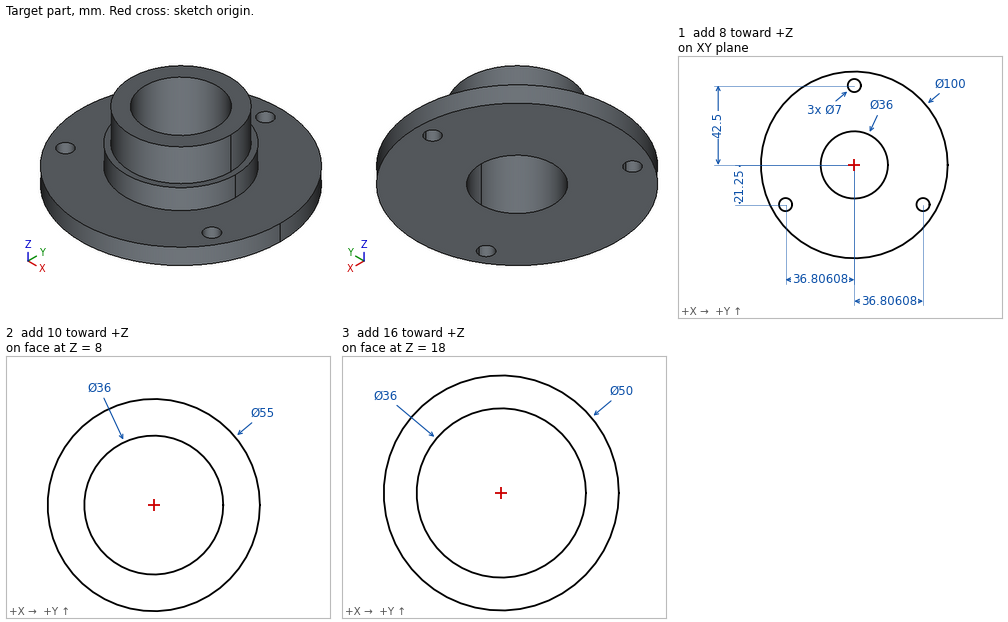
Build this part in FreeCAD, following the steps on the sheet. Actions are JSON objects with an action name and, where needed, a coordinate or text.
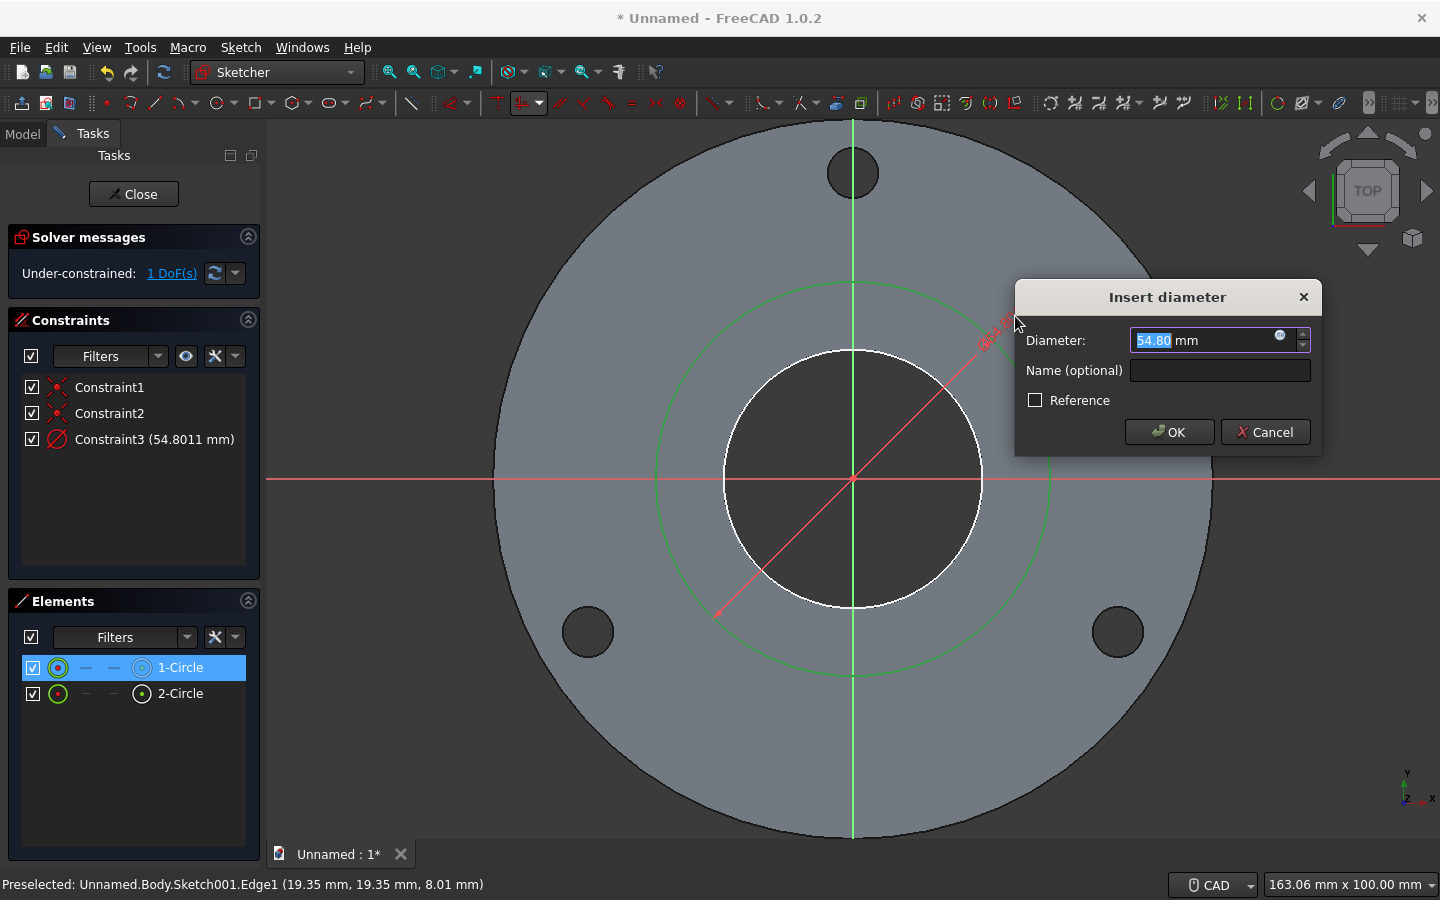
{"action": "type", "text": "55"}
{"action": "key", "text": "Return"}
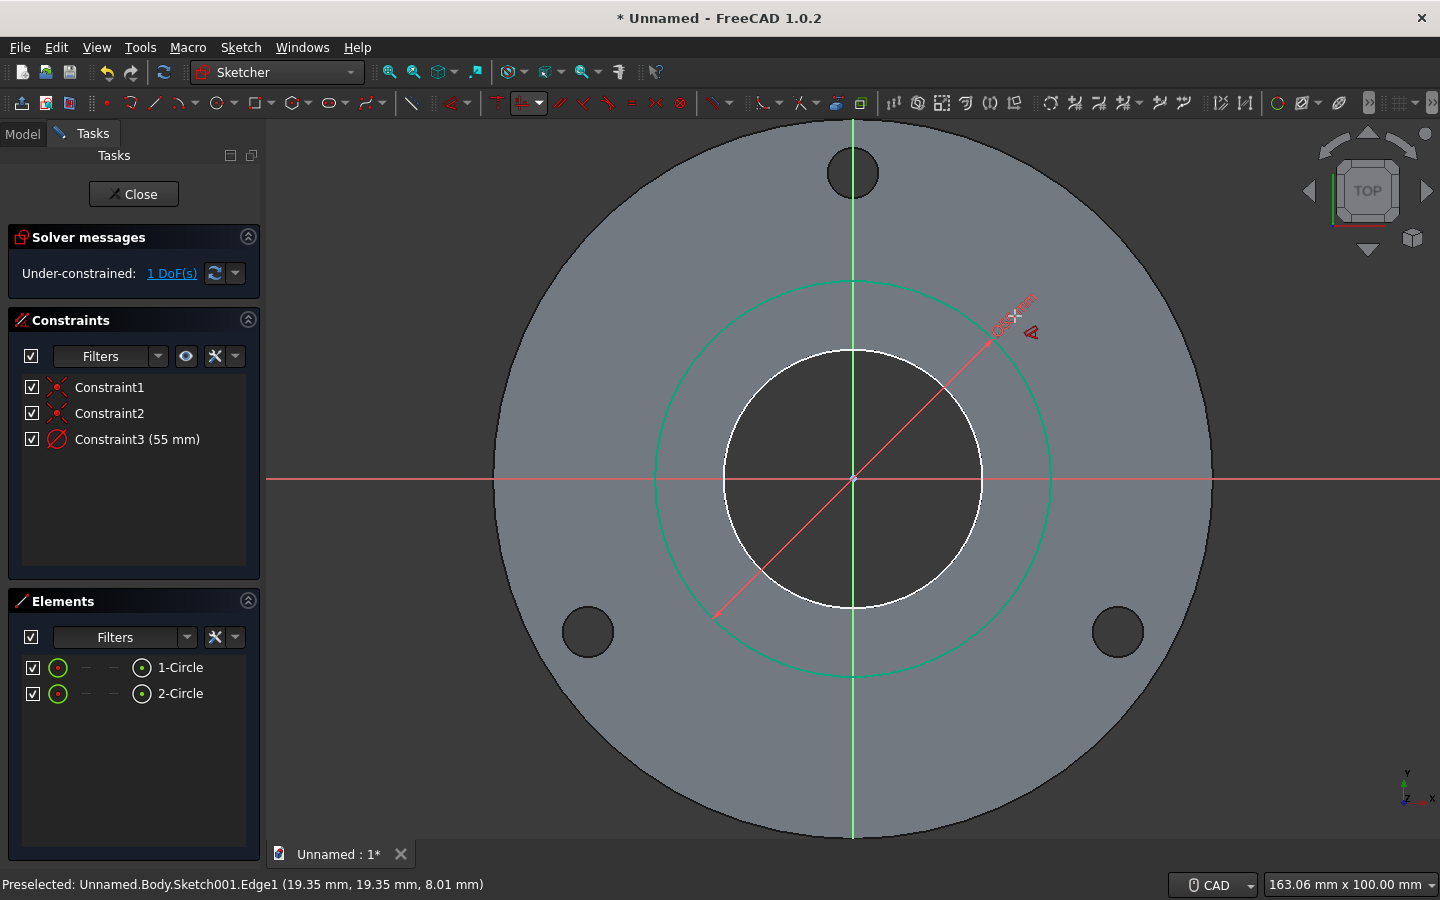
{"action": "left_click", "coordinate": [944, 387]}
{"action": "left_click", "coordinate": [967, 364]}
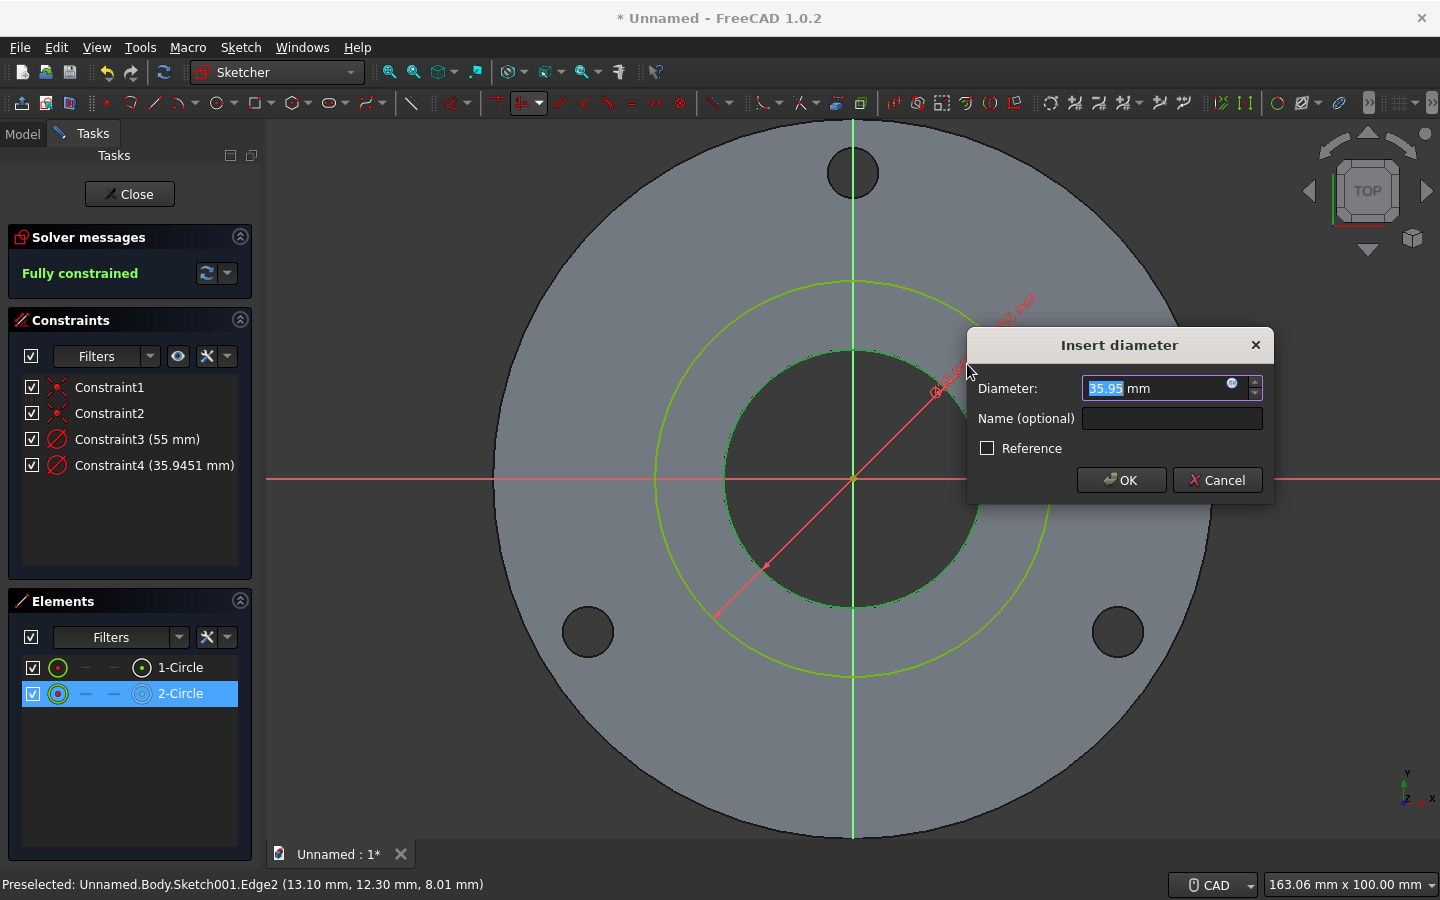
{"action": "type", "text": "36"}
{"action": "key", "text": "Return"}
{"action": "key", "text": "Escape"}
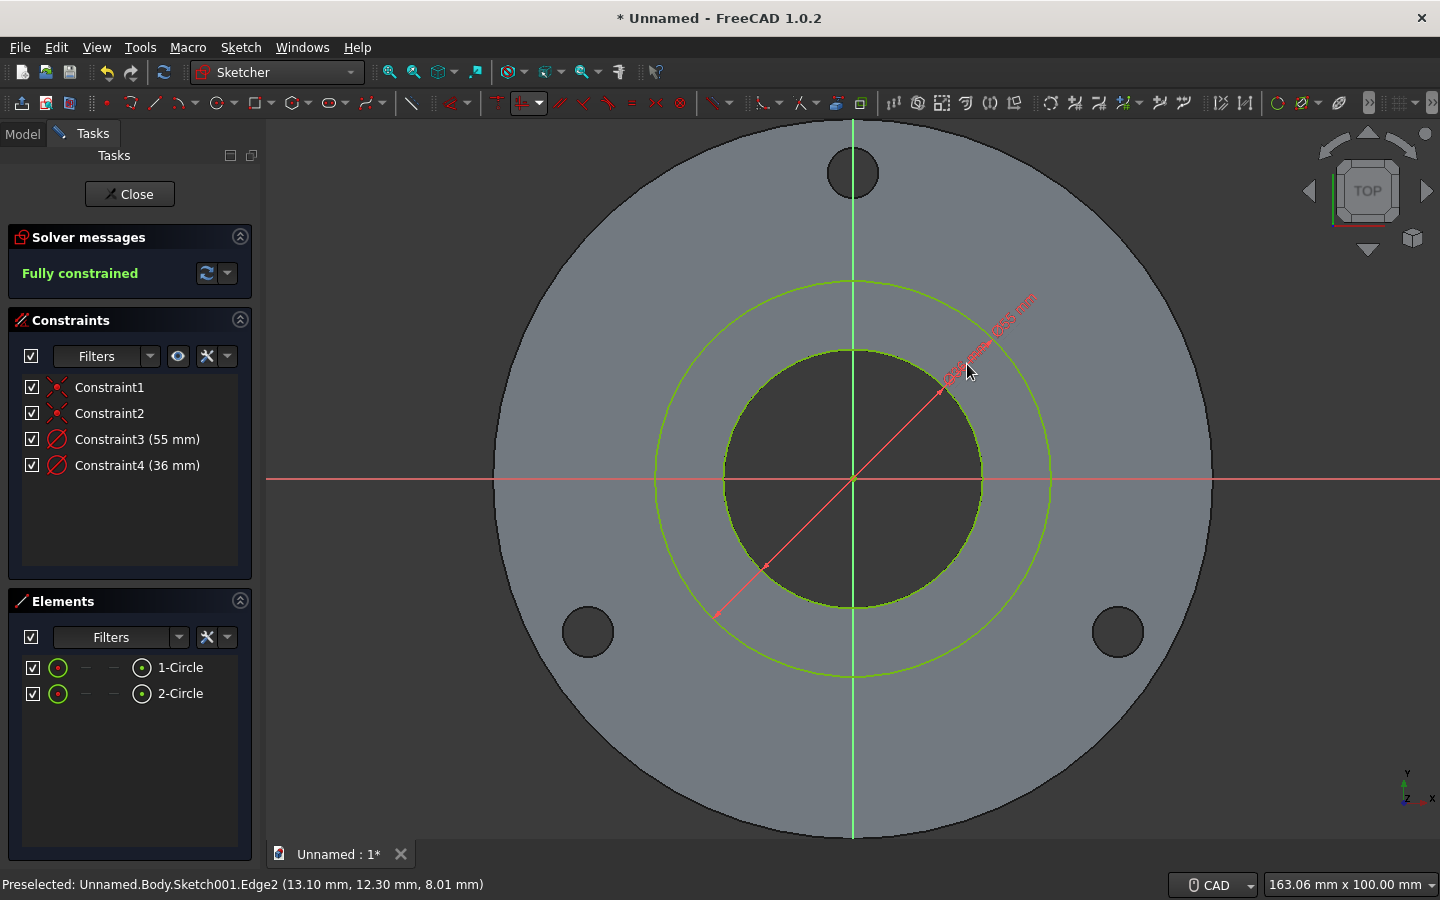
{"action": "left_click", "coordinate": [130, 194]}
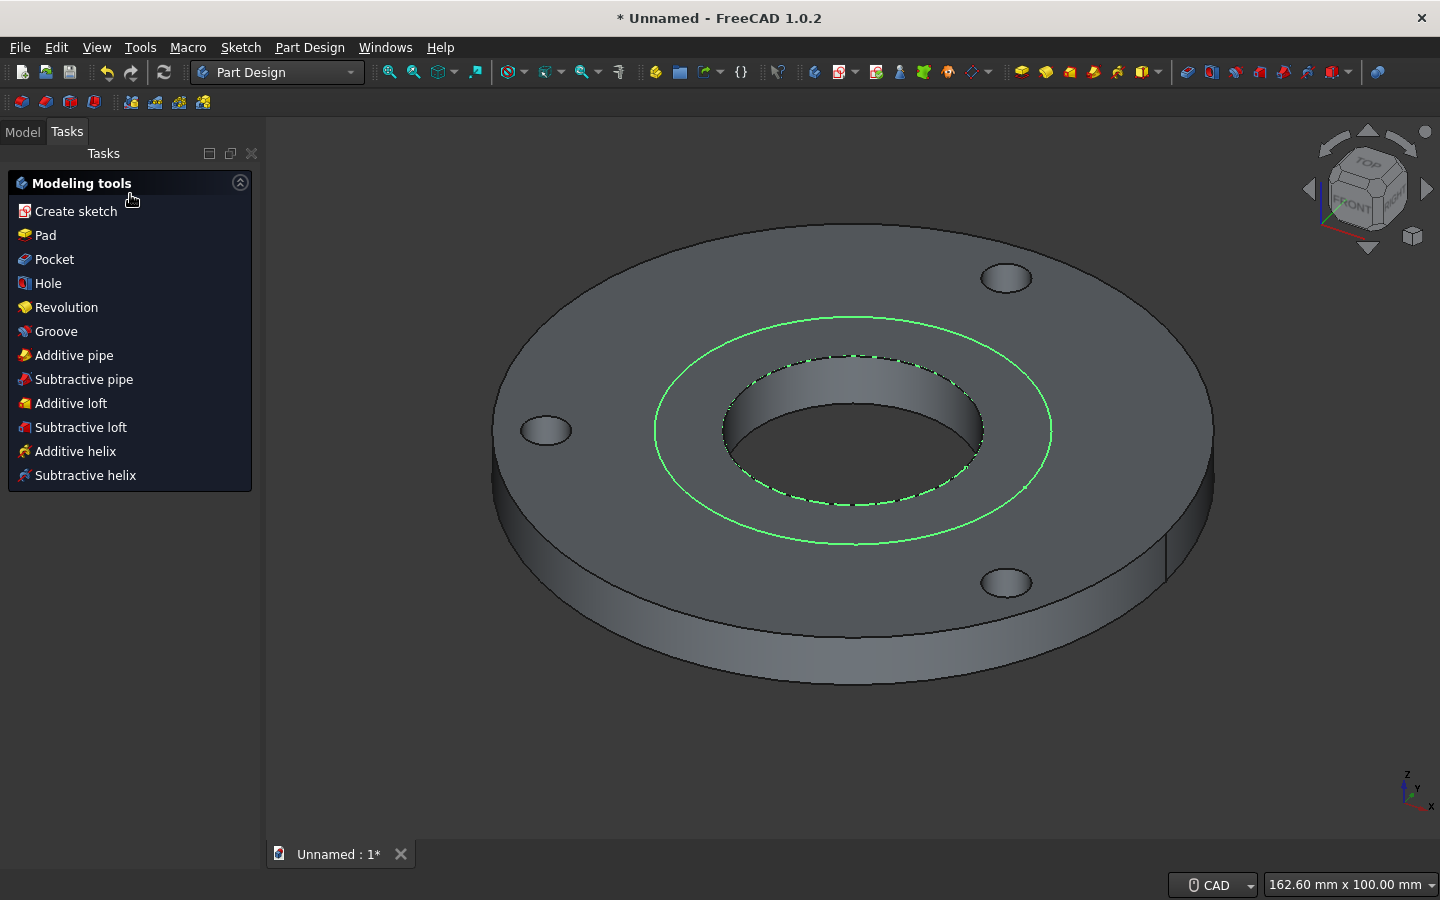
{"action": "left_click", "coordinate": [1022, 72]}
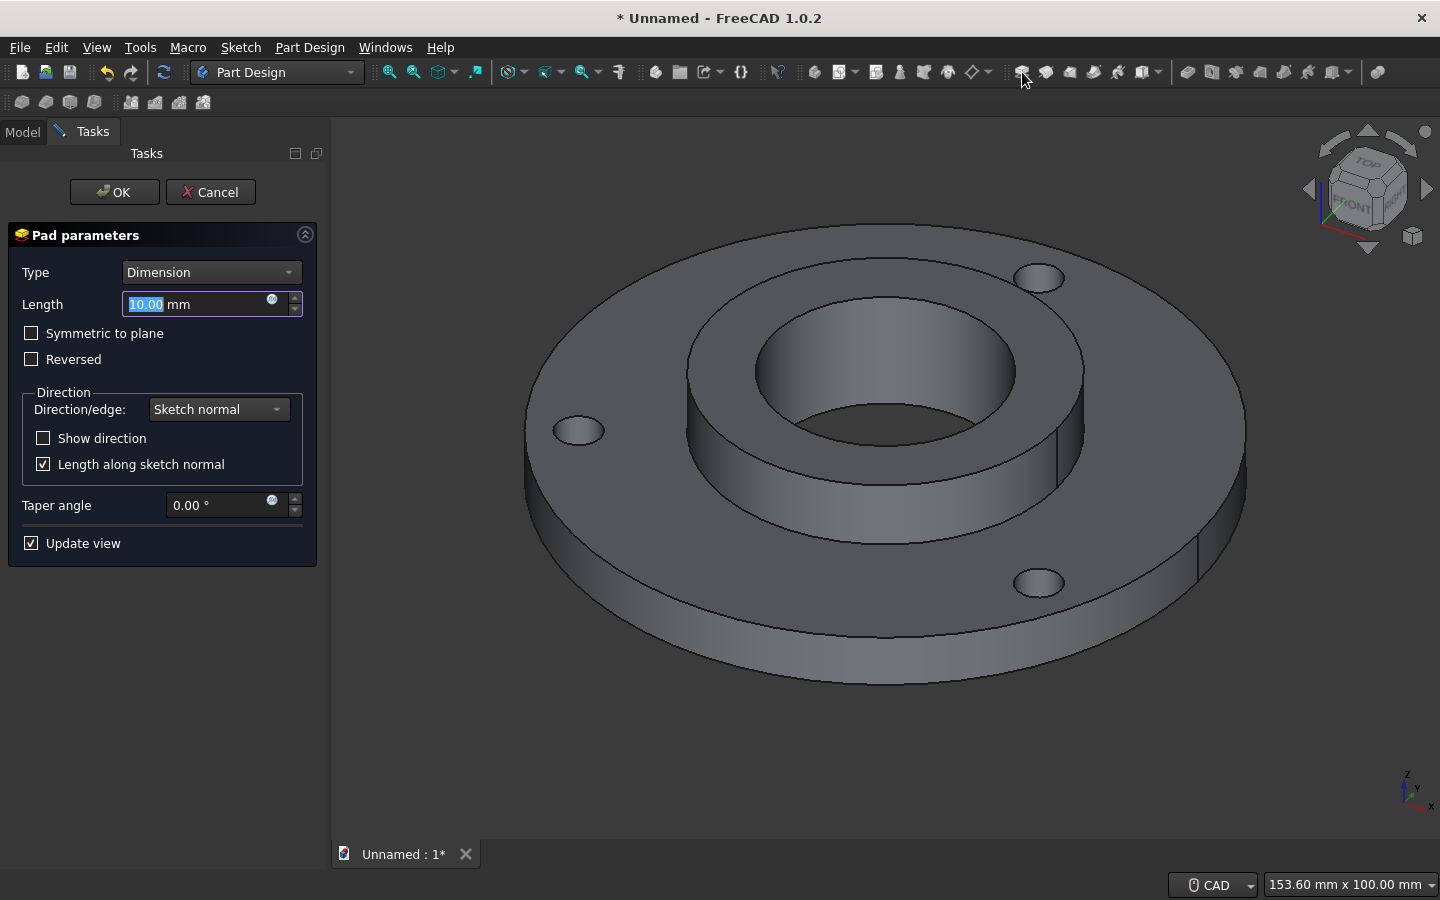
{"action": "type", "text": "10"}
{"action": "key", "text": "Tab"}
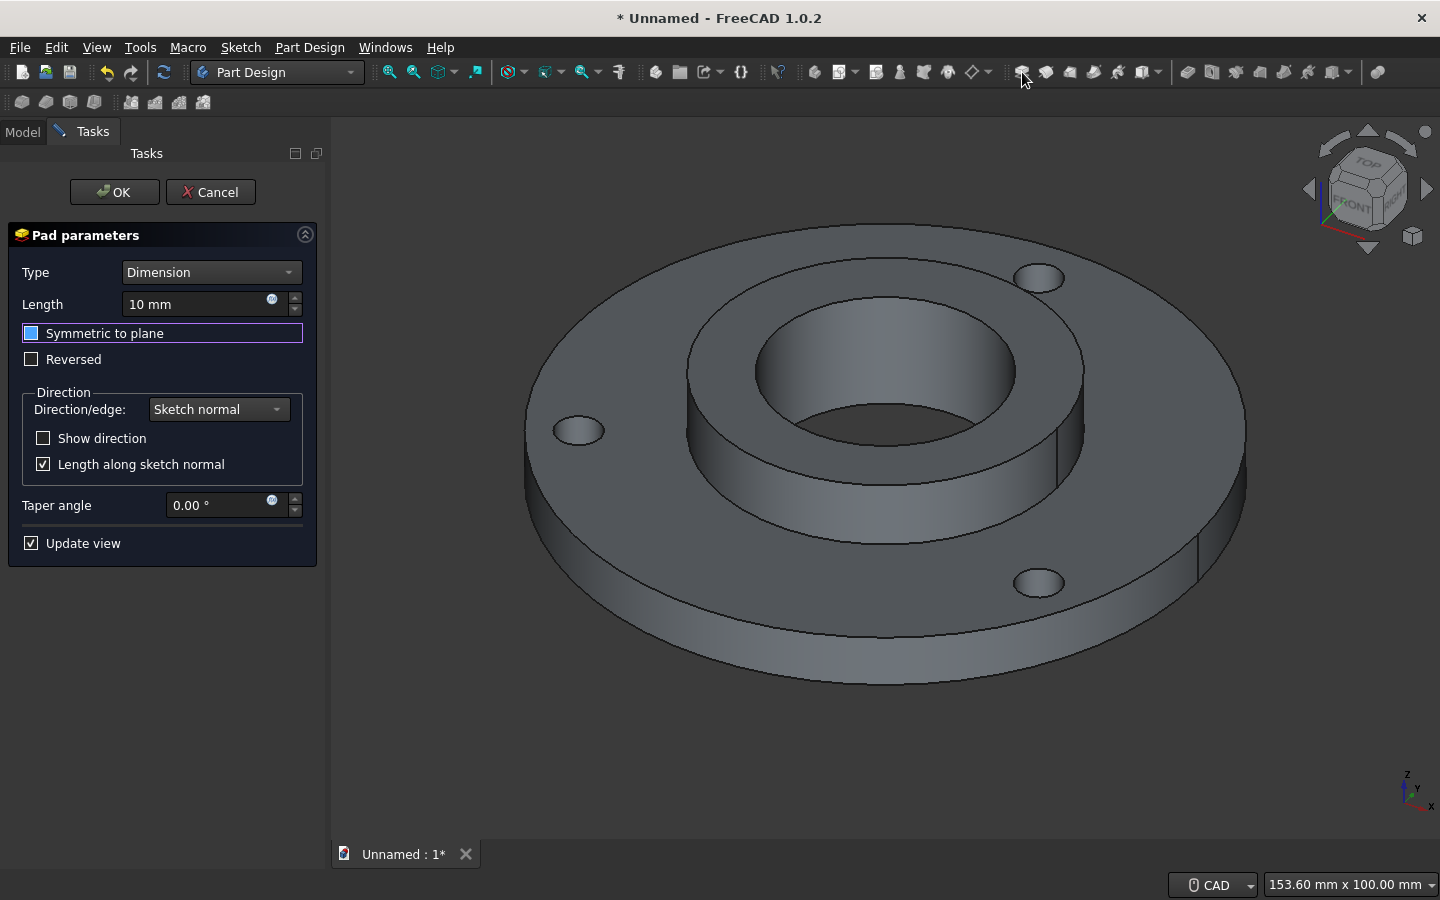
{"action": "left_click", "coordinate": [115, 192]}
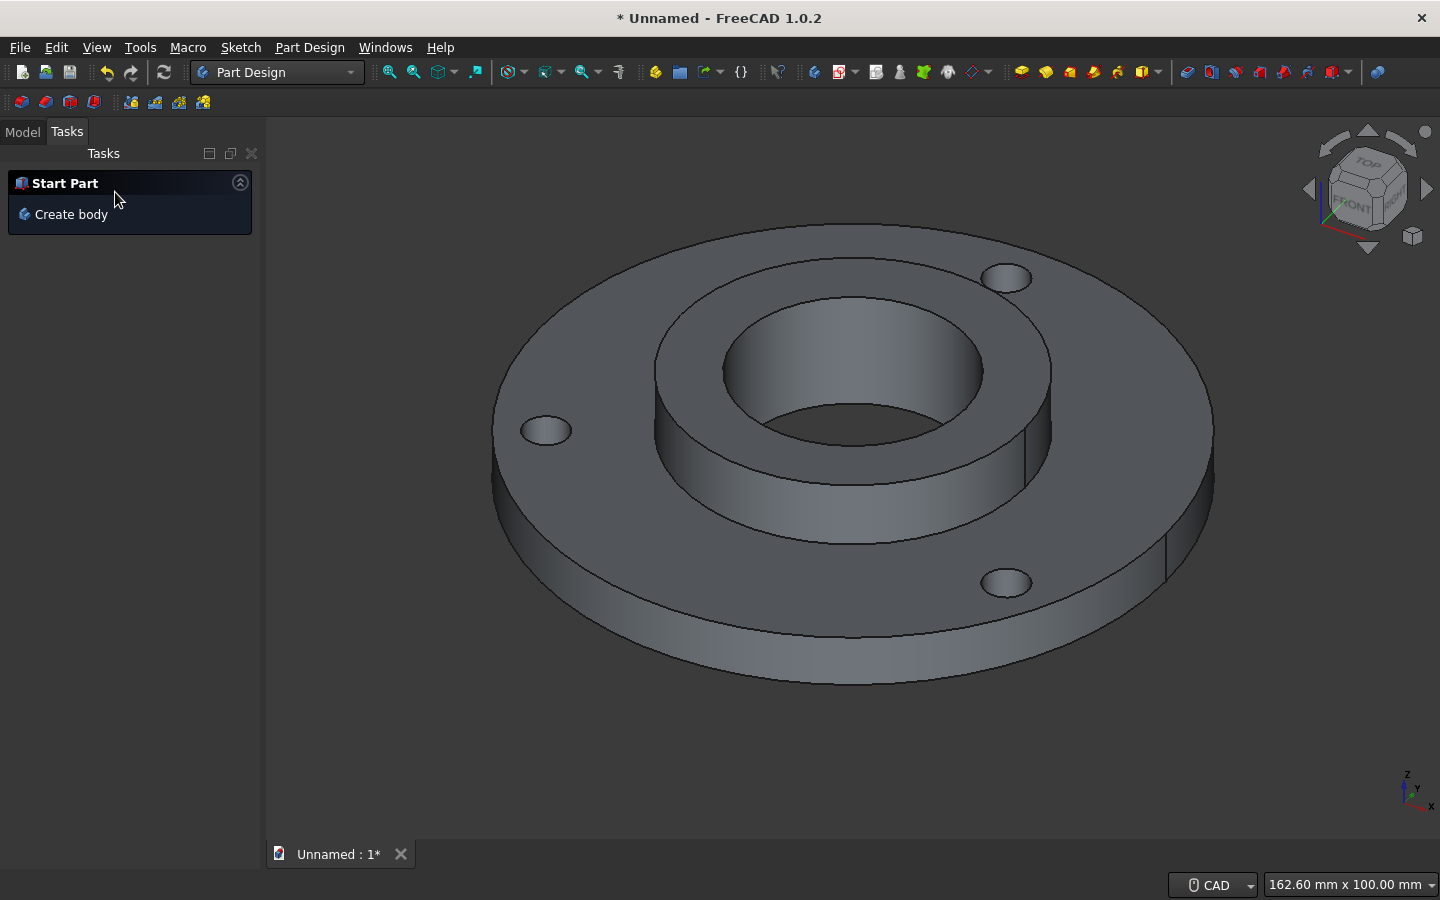
{"action": "left_click", "coordinate": [390, 72]}